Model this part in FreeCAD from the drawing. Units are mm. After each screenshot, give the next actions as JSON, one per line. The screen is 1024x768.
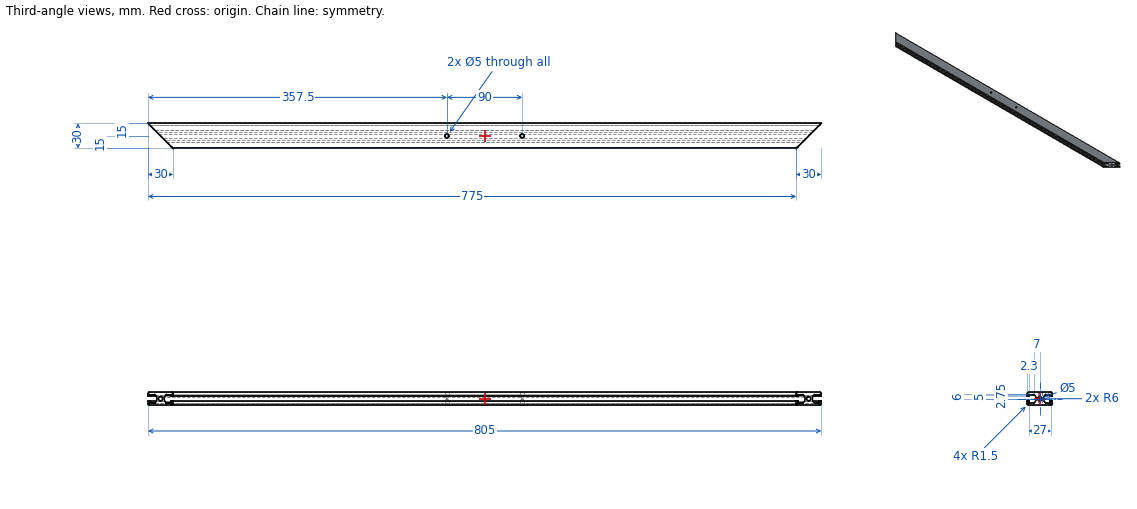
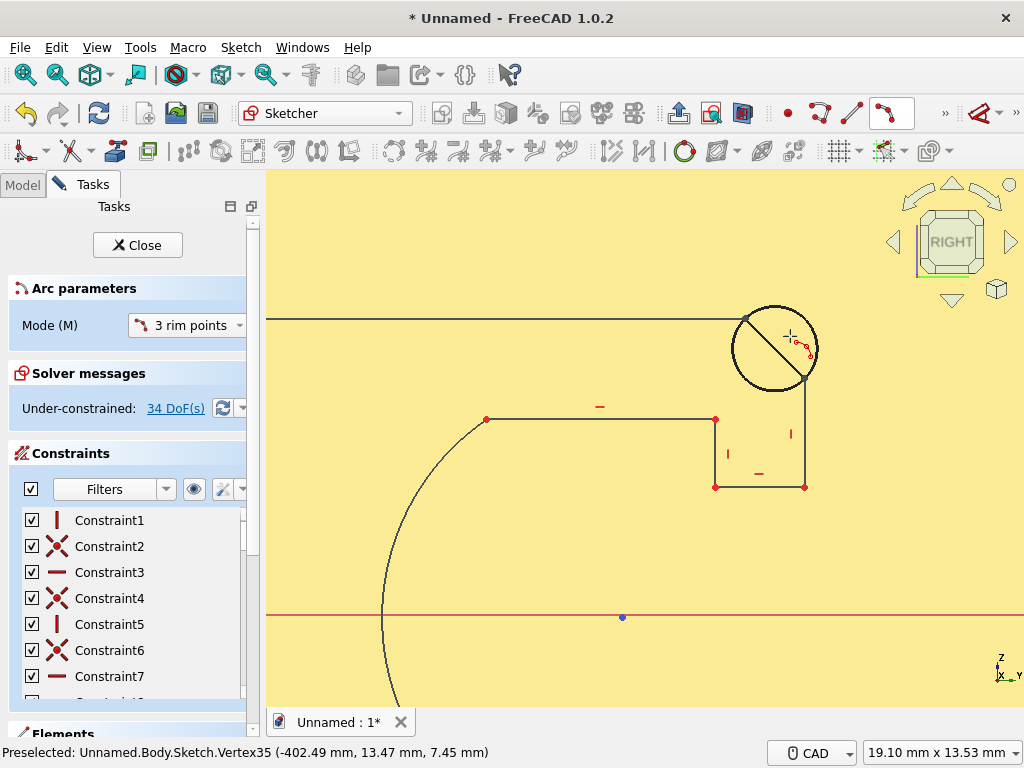
{"action": "left_click", "coordinate": [788, 334]}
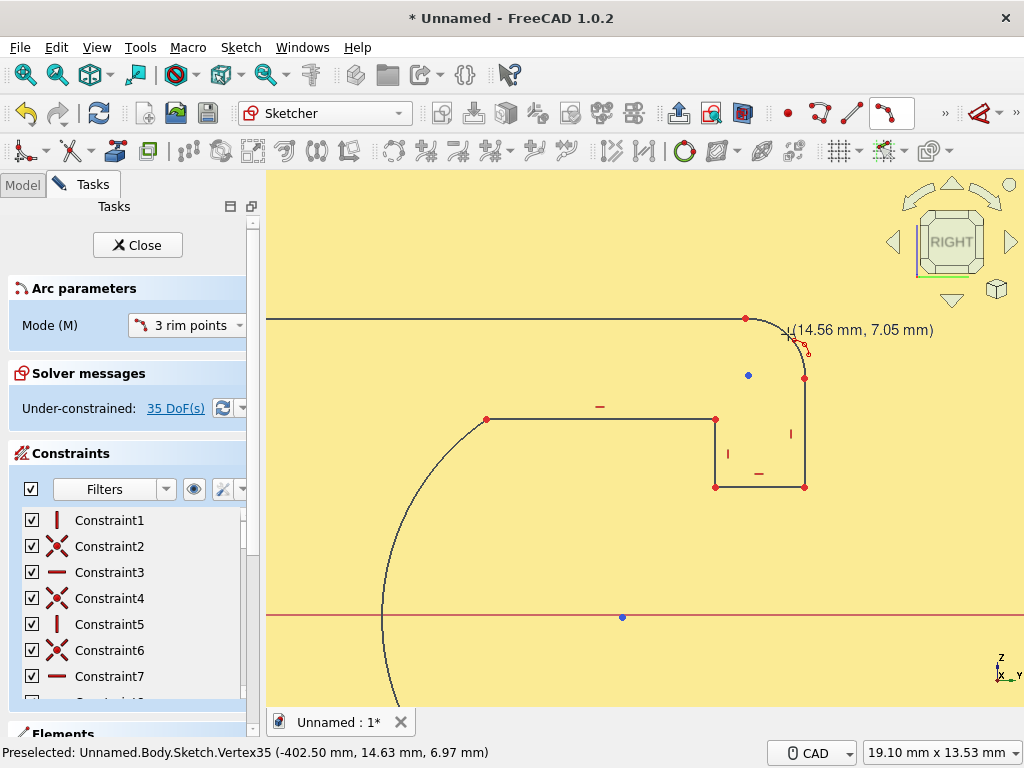
{"action": "scroll", "coordinate": [790, 336], "scroll_direction": "down", "scroll_amount": 5}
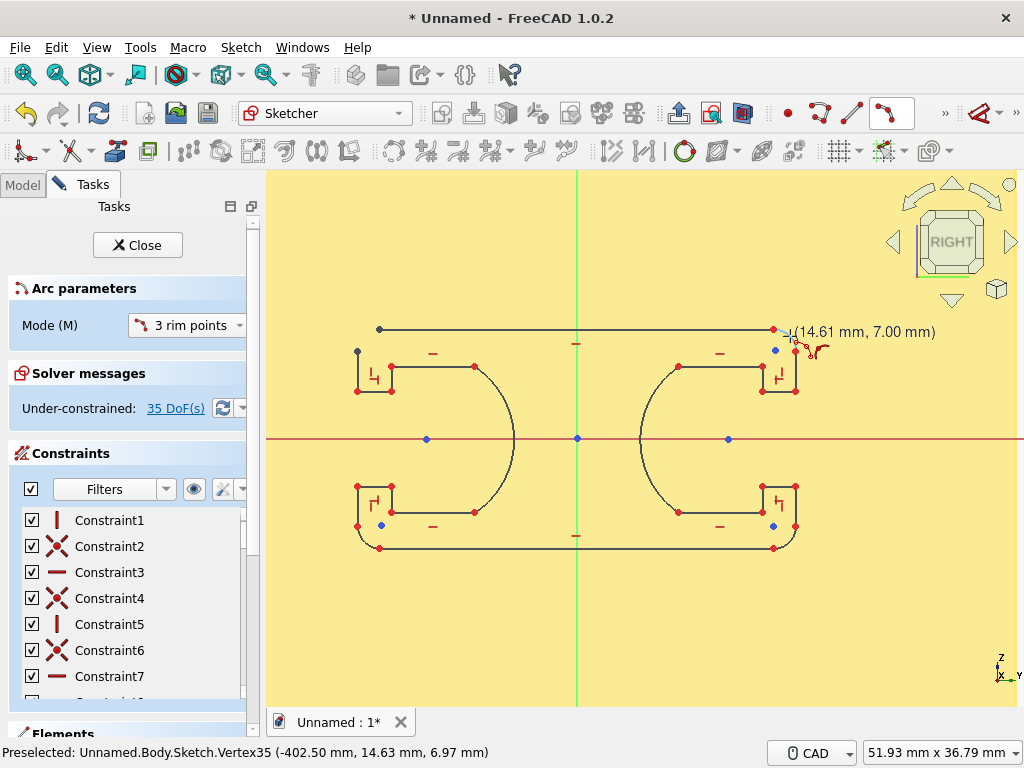
{"action": "left_click", "coordinate": [380, 330]}
{"action": "left_click", "coordinate": [358, 352]}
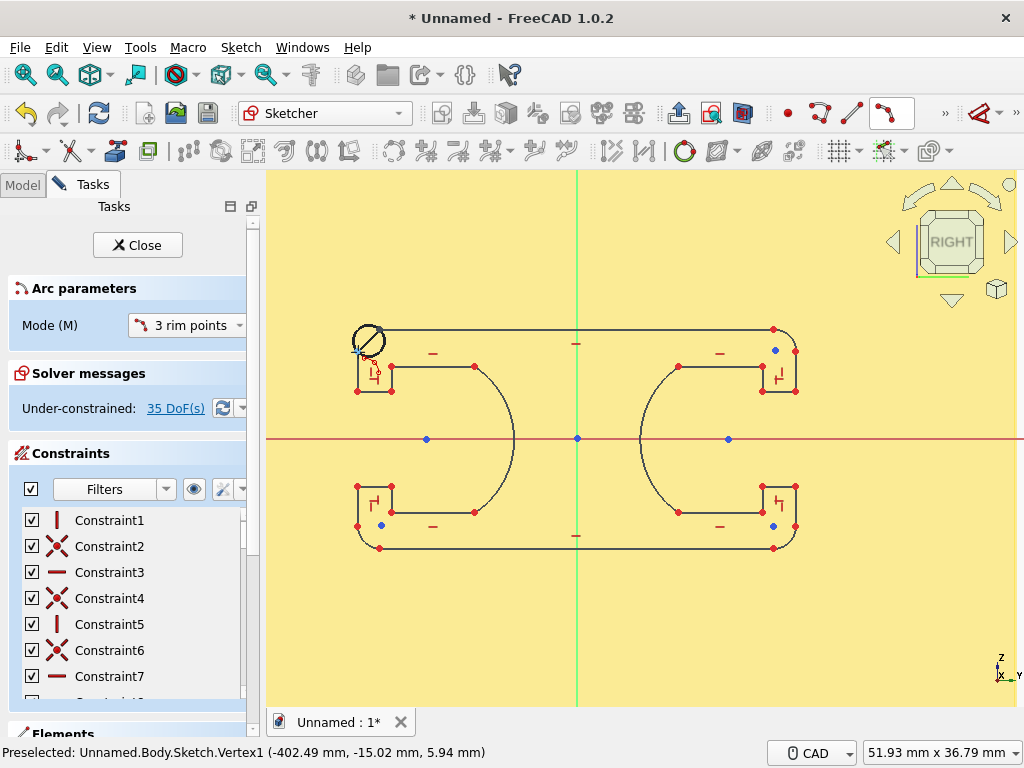
{"action": "scroll", "coordinate": [365, 336], "scroll_direction": "up", "scroll_amount": 5}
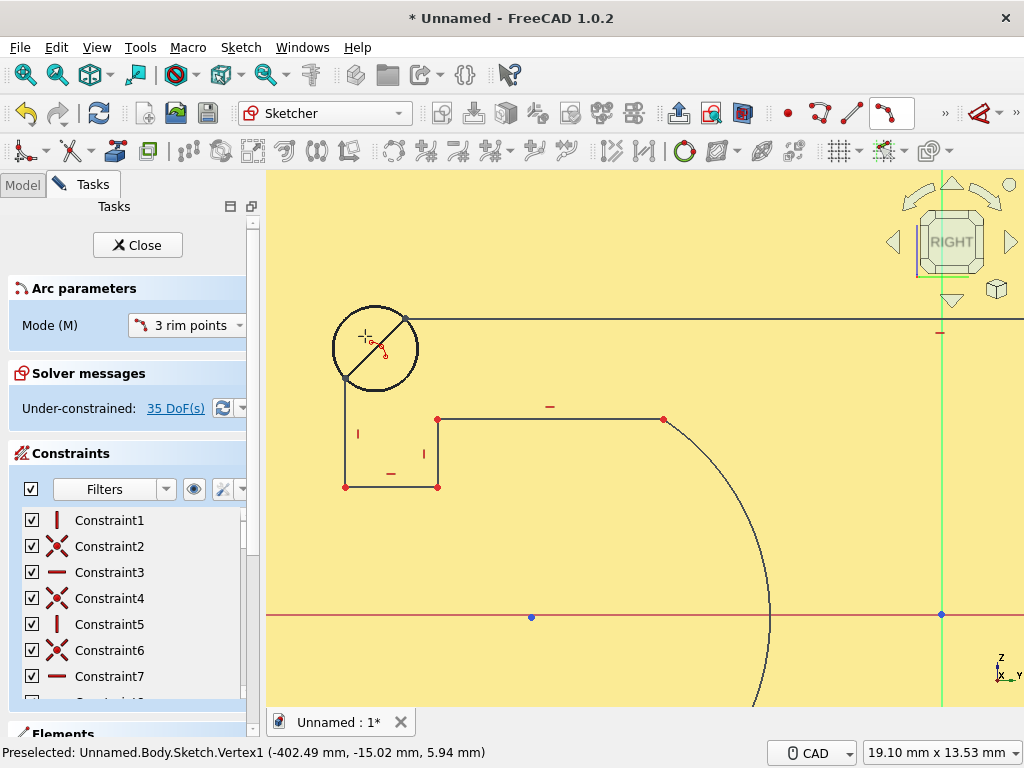
{"action": "left_click", "coordinate": [364, 334]}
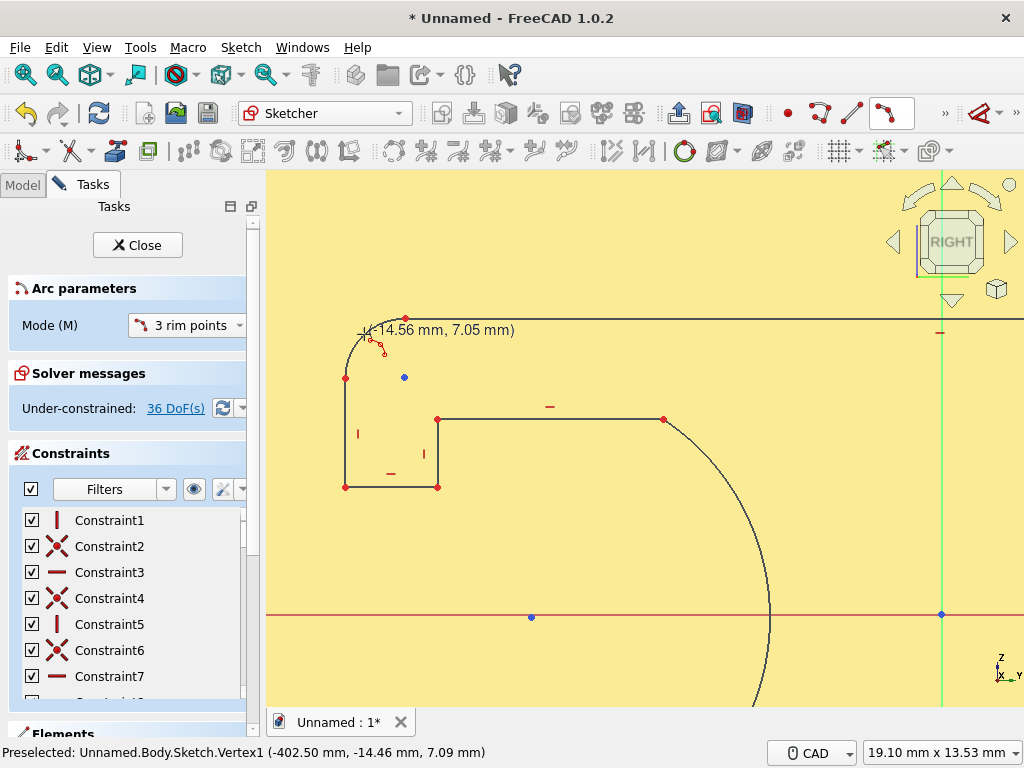
{"action": "key", "text": "g c"}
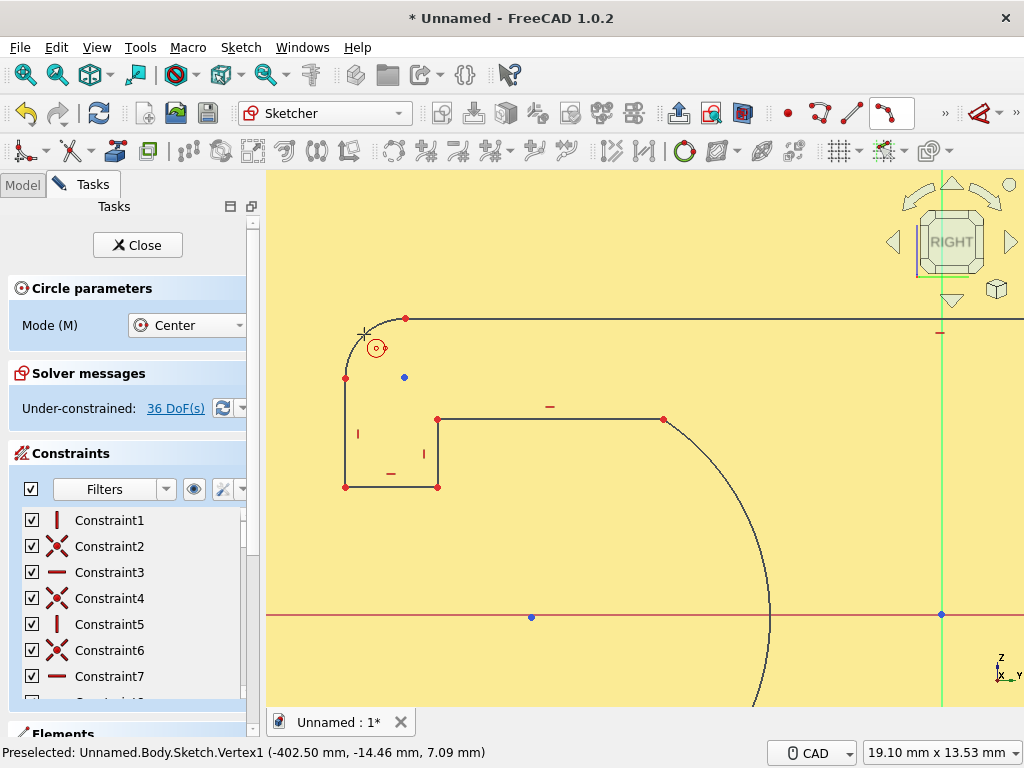
{"action": "scroll", "coordinate": [364, 336], "scroll_direction": "down", "scroll_amount": 5}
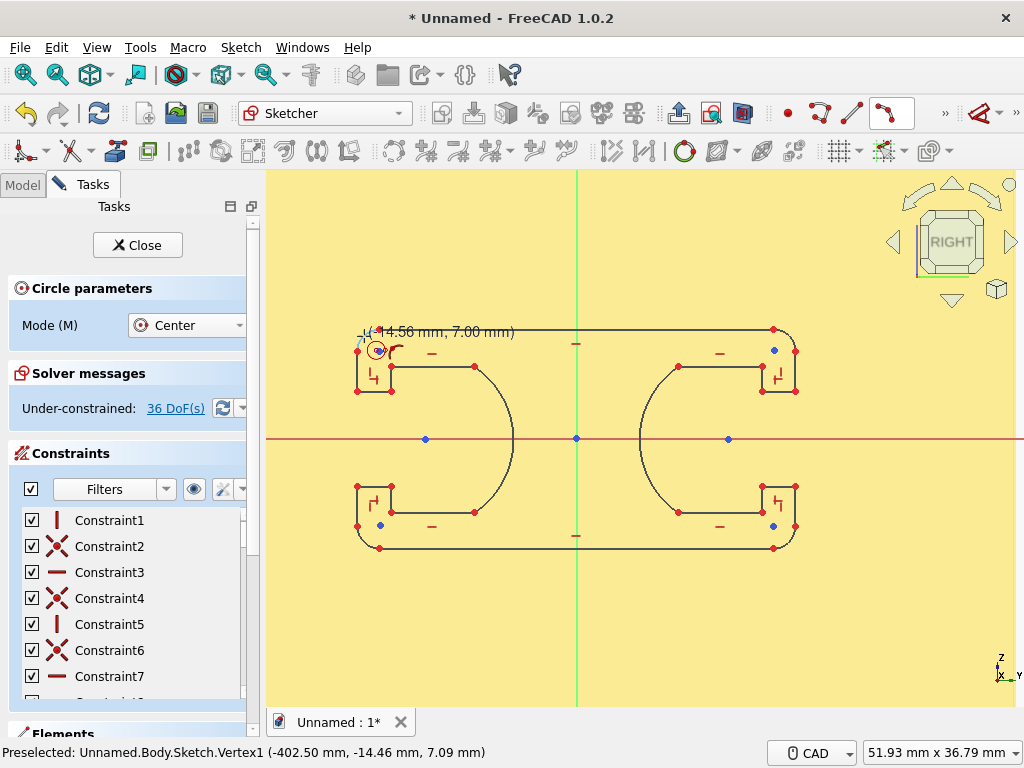
{"action": "left_click", "coordinate": [577, 439]}
{"action": "mouse_move", "coordinate": [602, 413]}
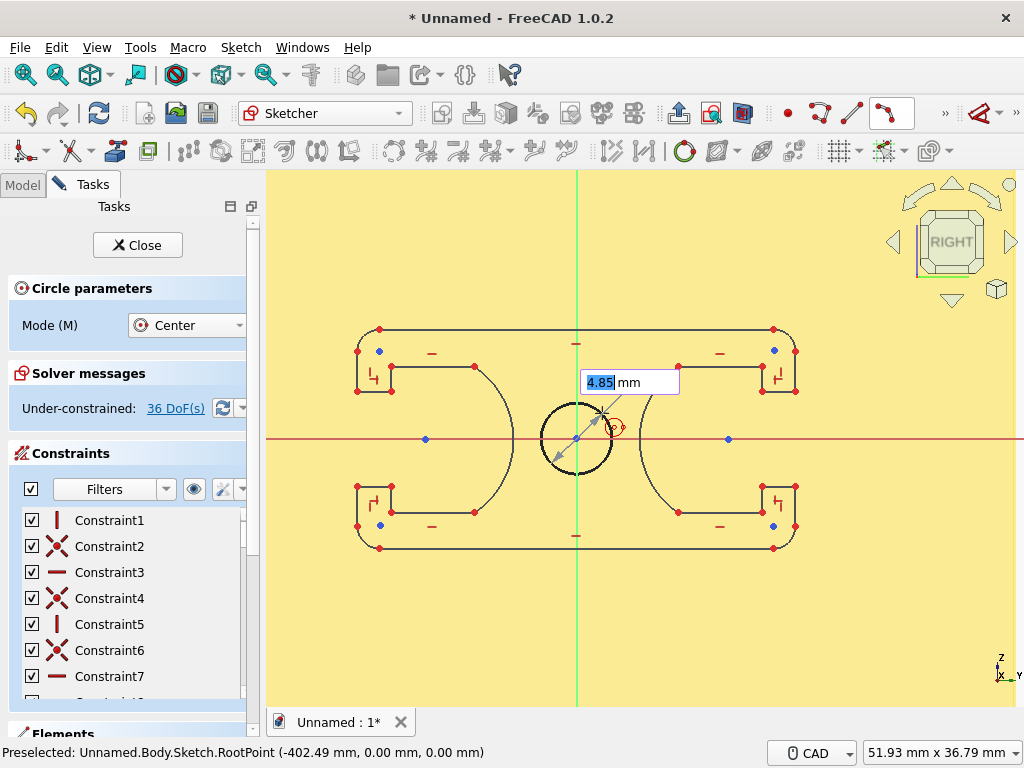
{"action": "type", "text": "5"}
{"action": "key", "text": "Return"}
{"action": "key", "text": "Escape"}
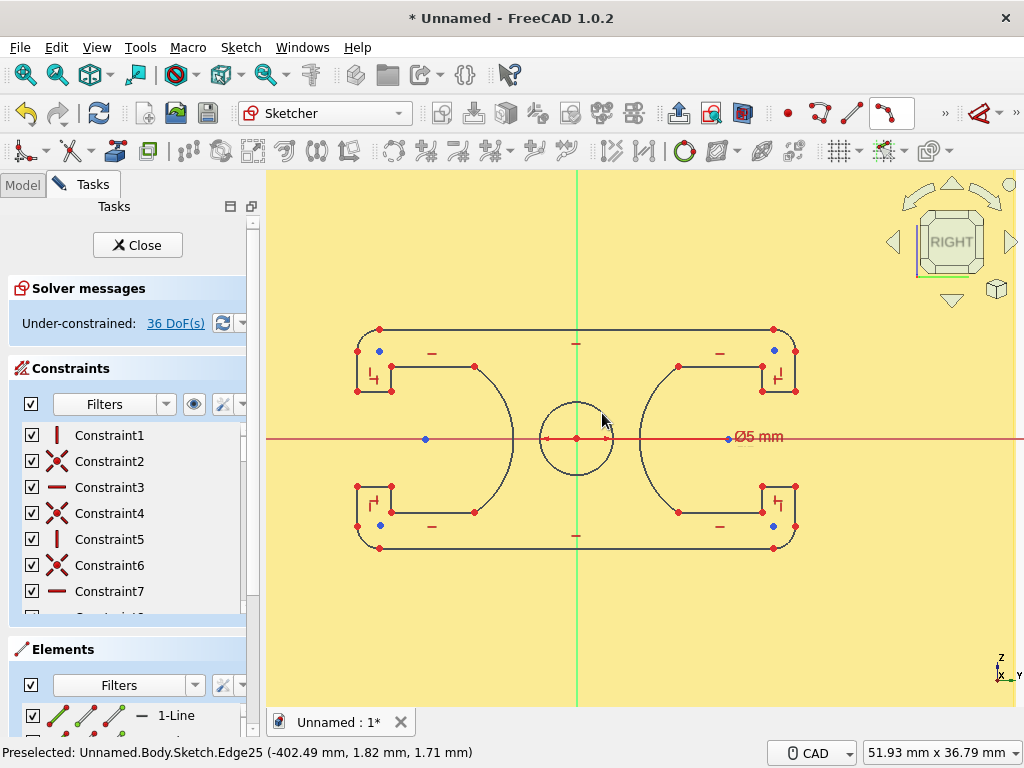
{"action": "left_click", "coordinate": [357, 364]}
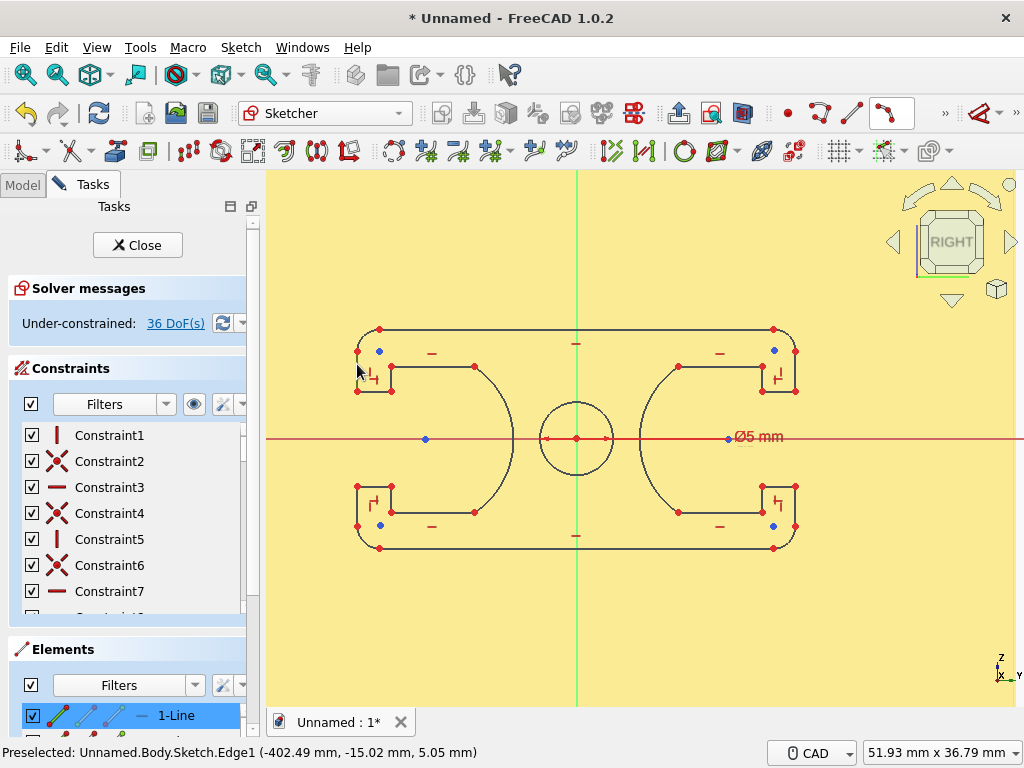
{"action": "scroll", "coordinate": [369, 332], "scroll_direction": "up", "scroll_amount": 2}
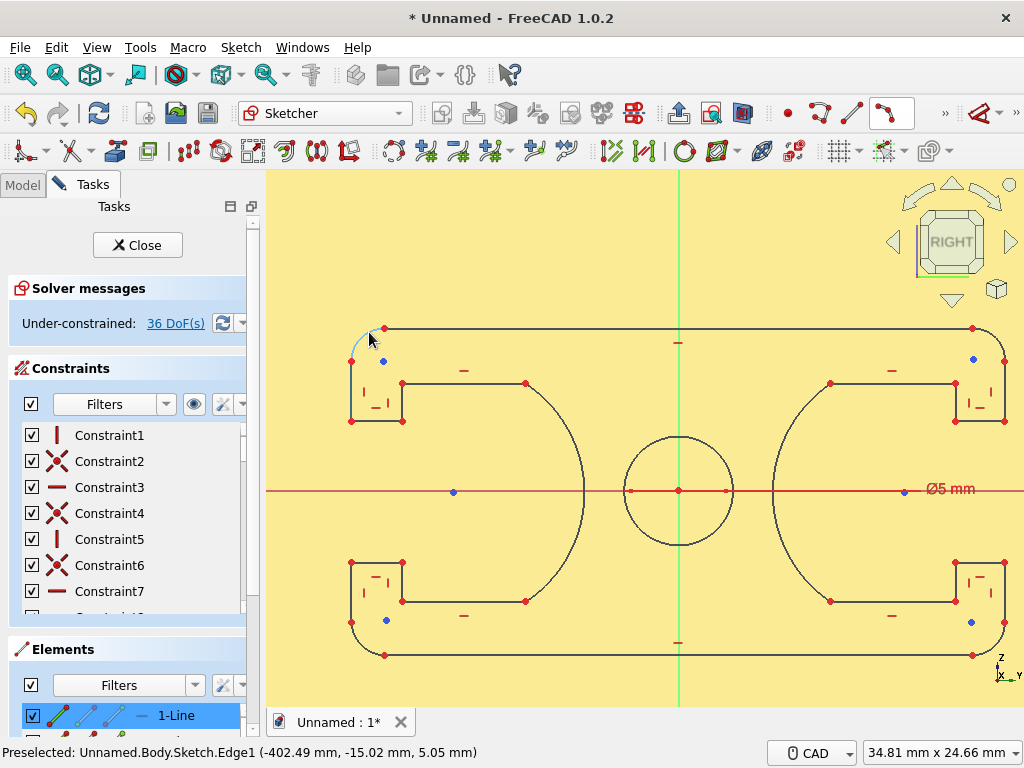
{"action": "left_click", "coordinate": [369, 332]}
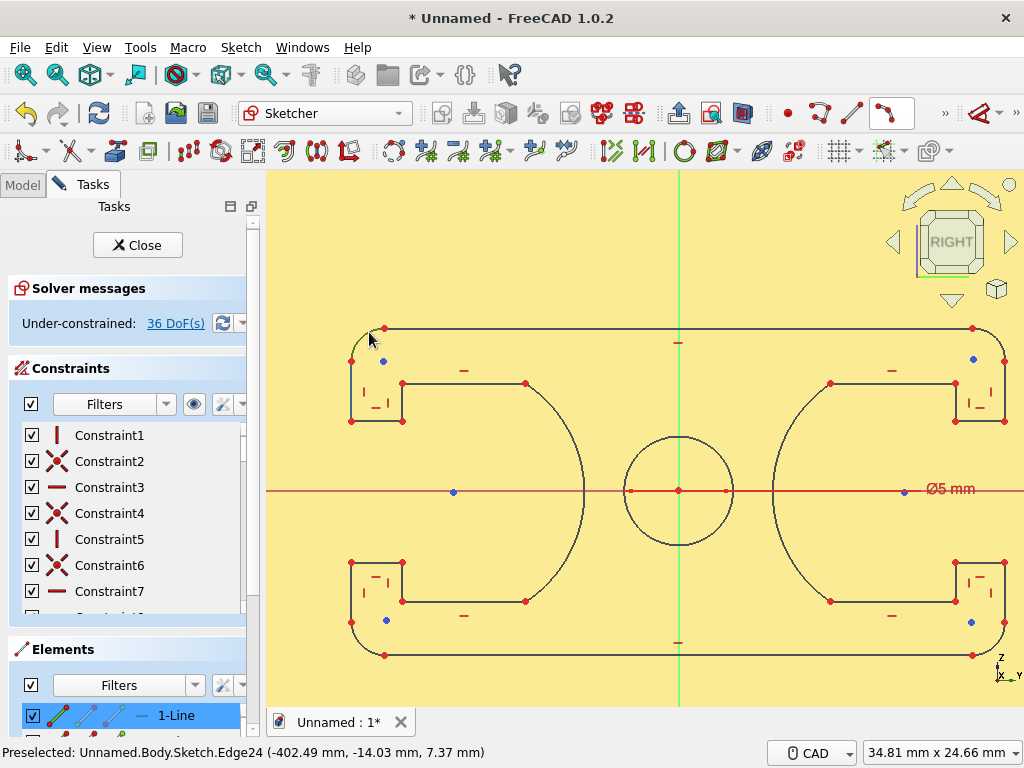
{"action": "key", "text": "t"}